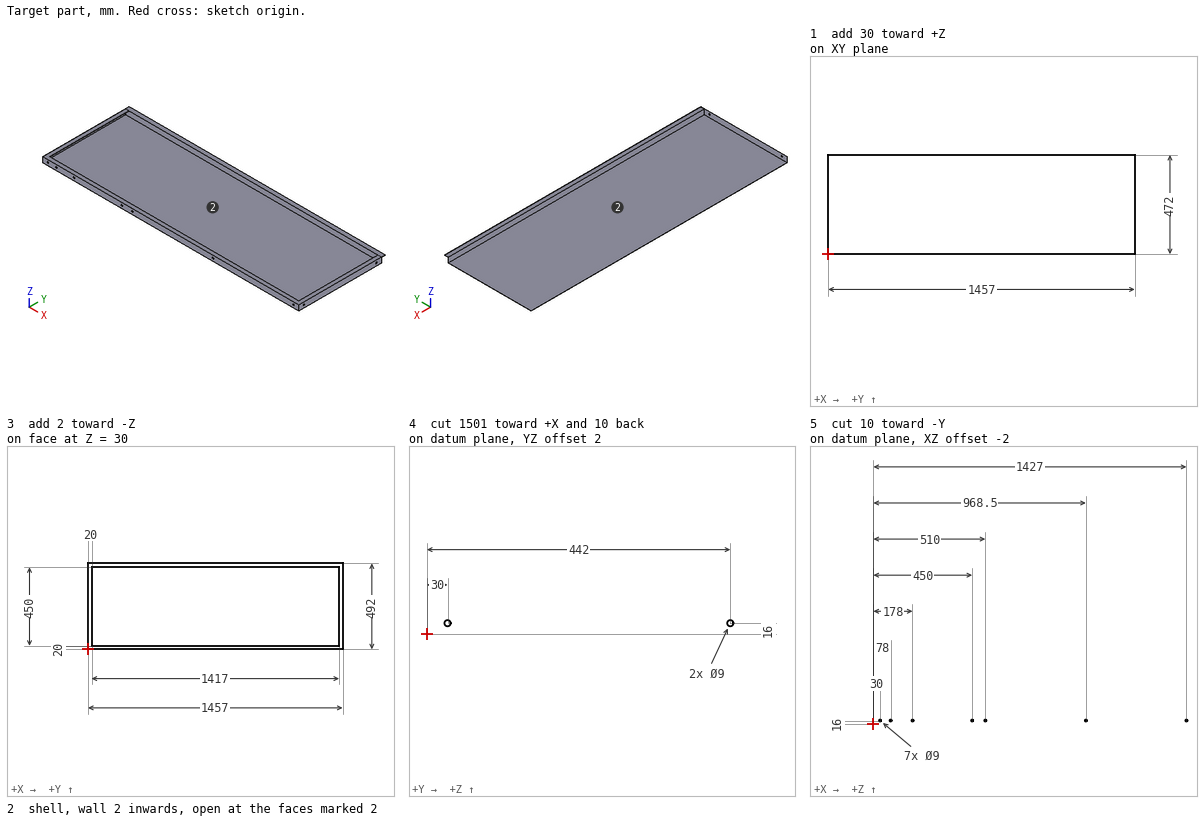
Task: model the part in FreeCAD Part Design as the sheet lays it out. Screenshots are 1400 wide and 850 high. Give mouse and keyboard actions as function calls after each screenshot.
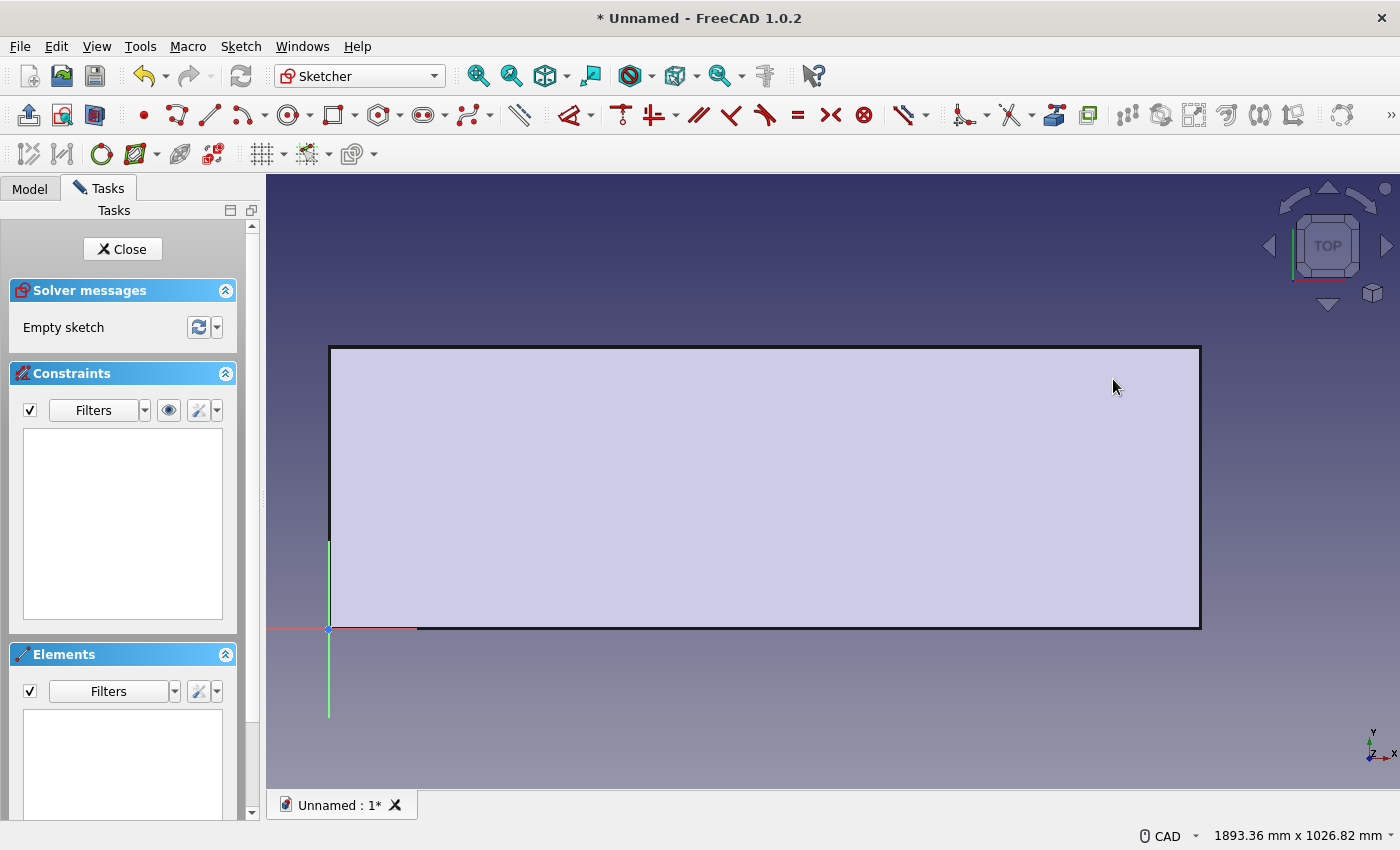
click(332, 116)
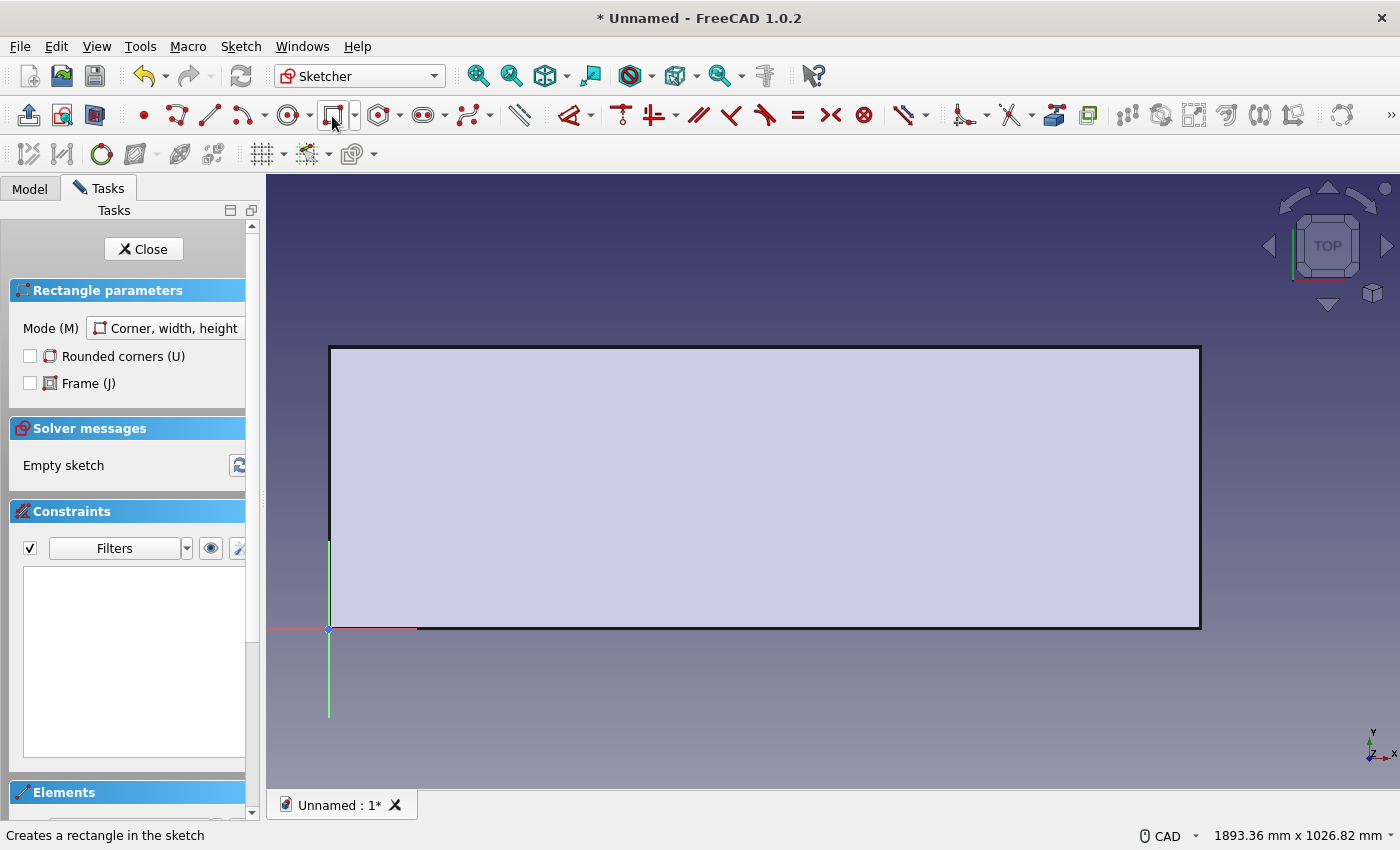
click(329, 629)
move(1201, 334)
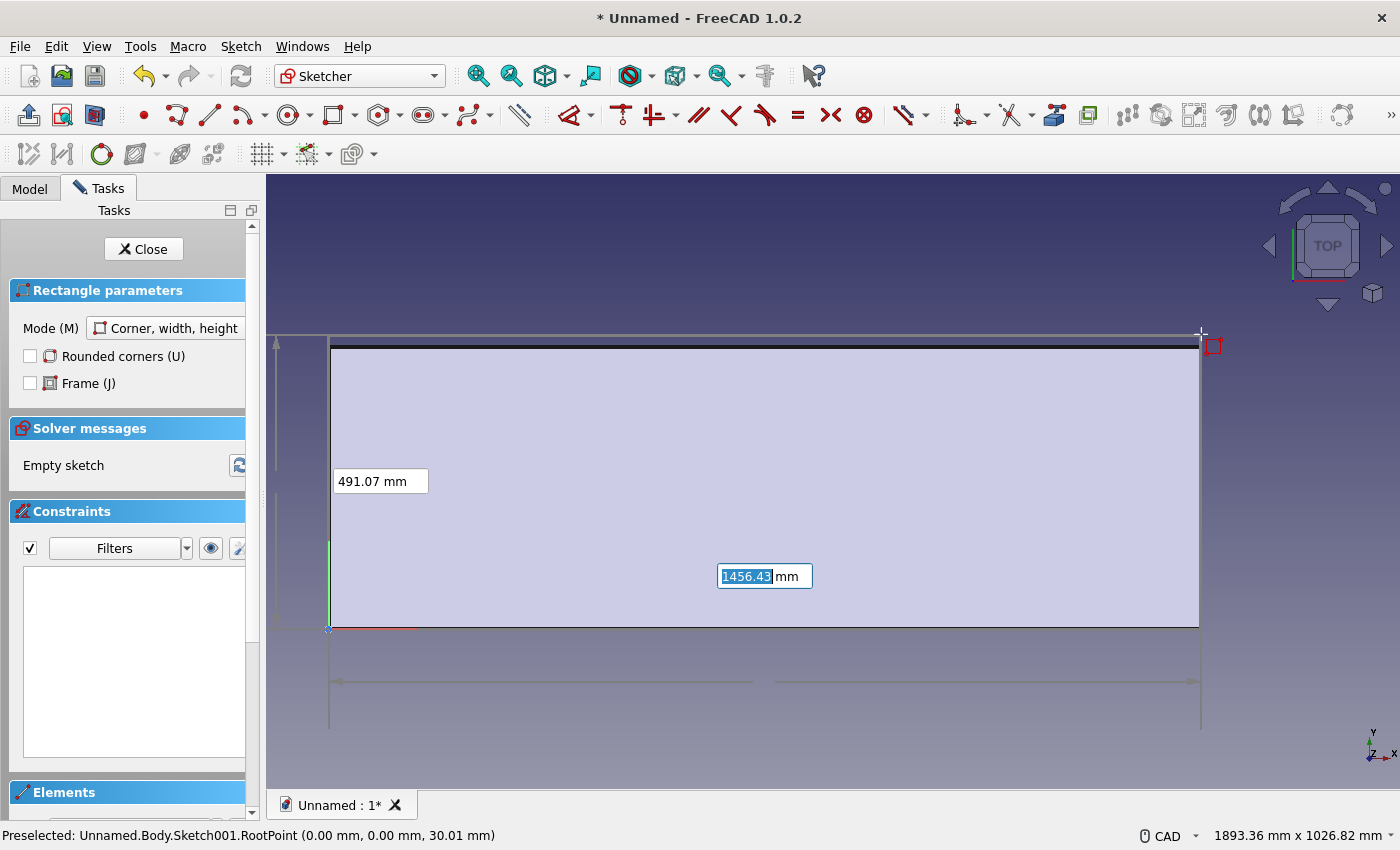
text(1457)
key(Tab)
text(492)
key(Return)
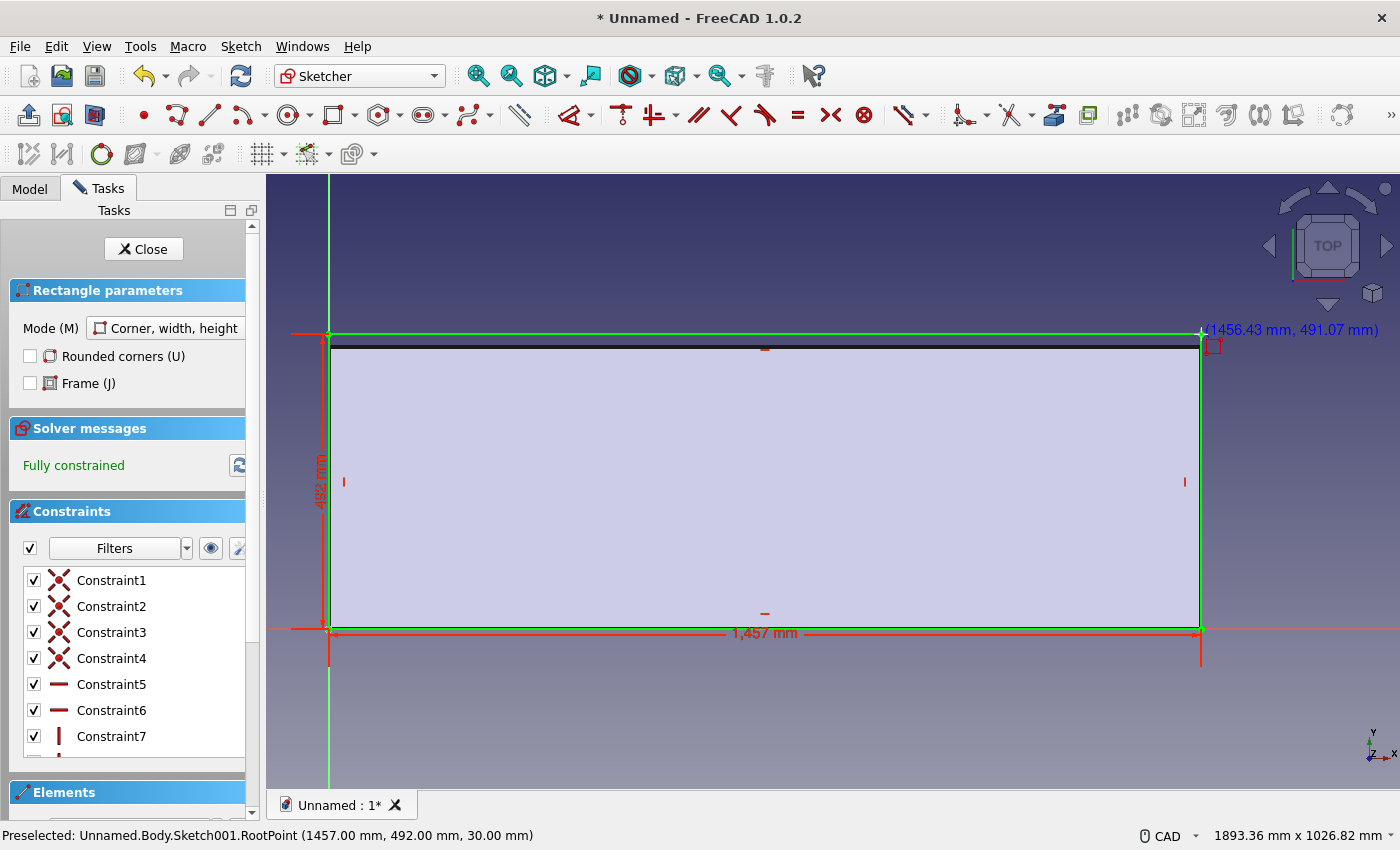
scroll(341, 348, up, 2)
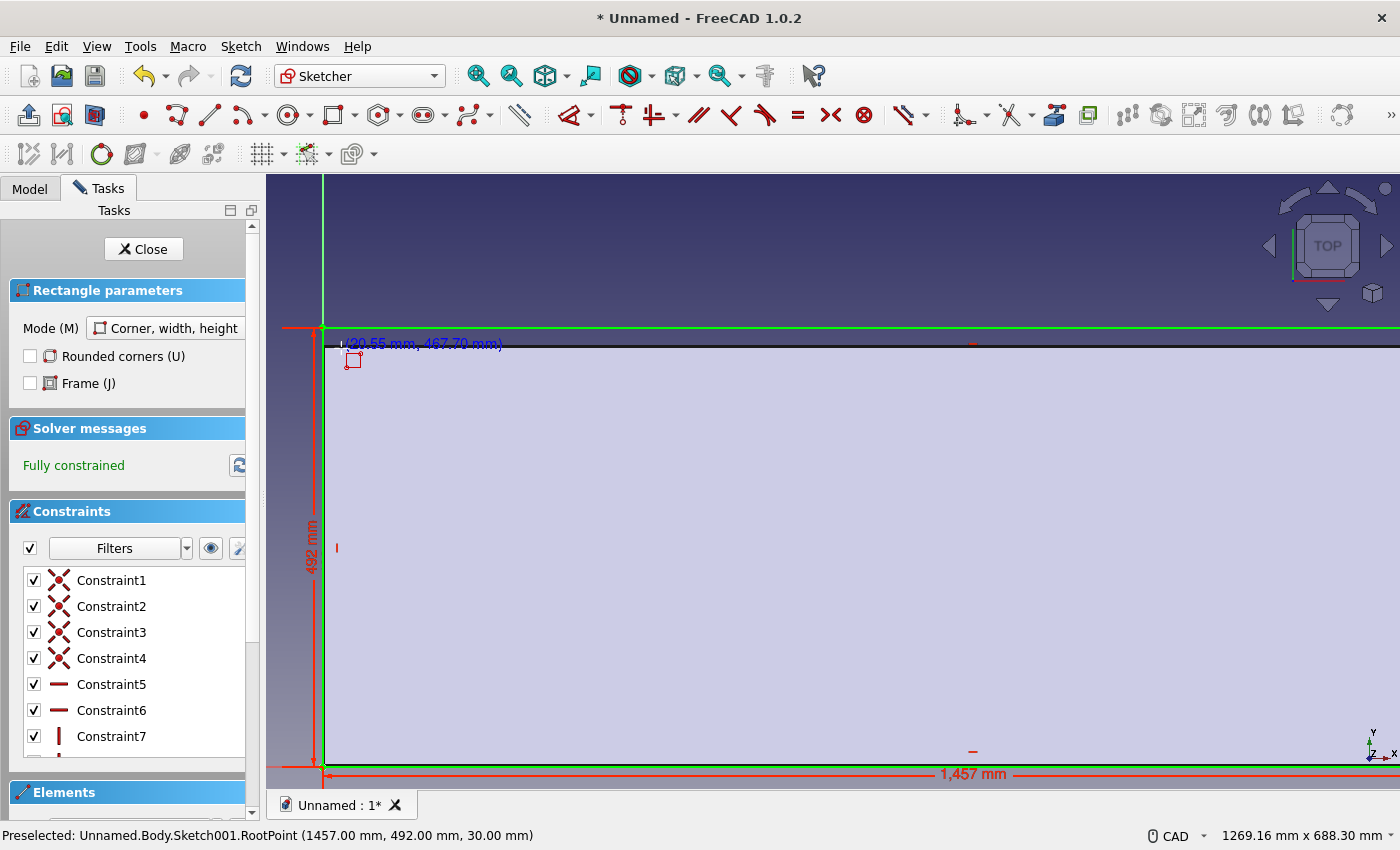
click(340, 347)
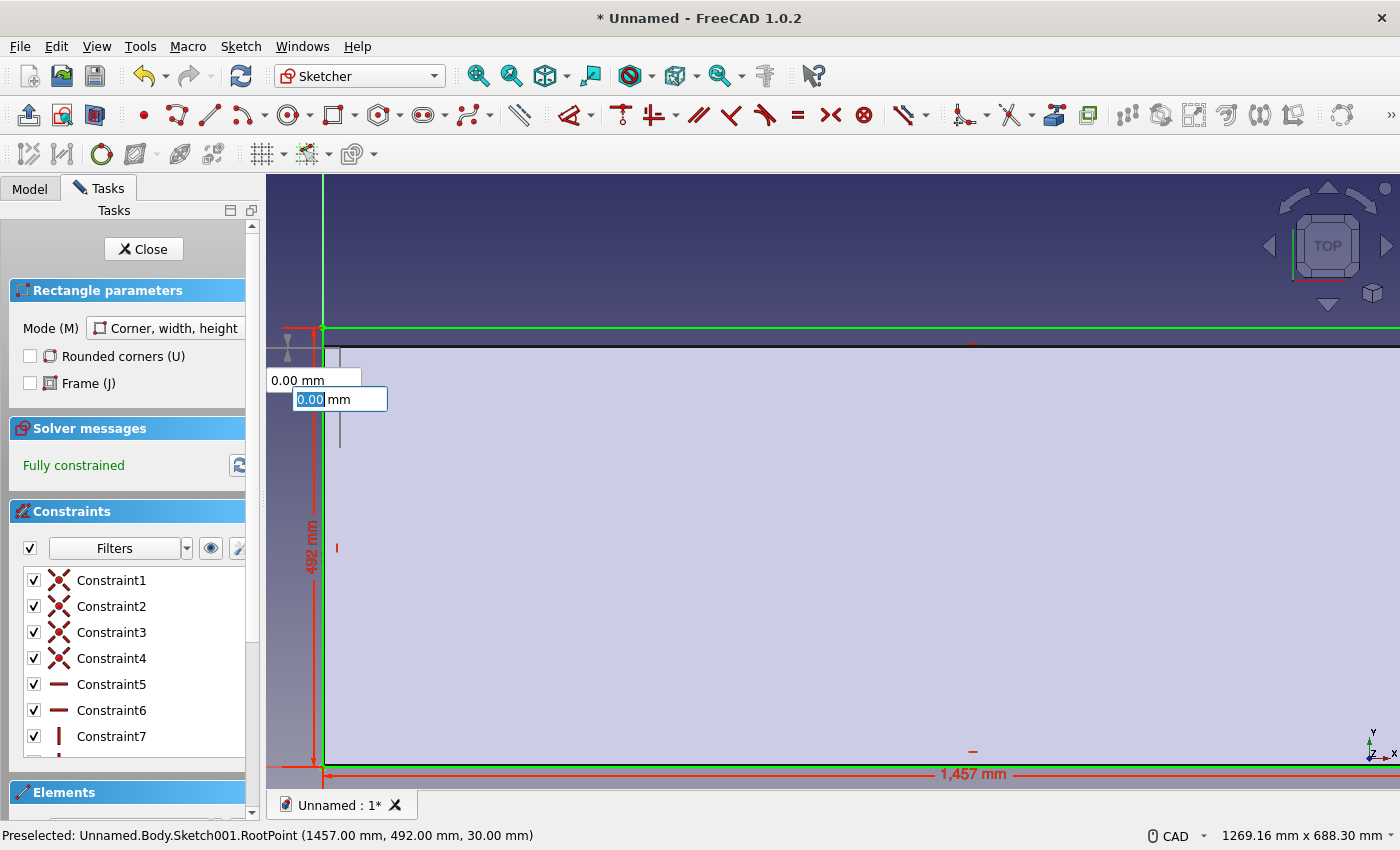
scroll(510, 401, down, 3)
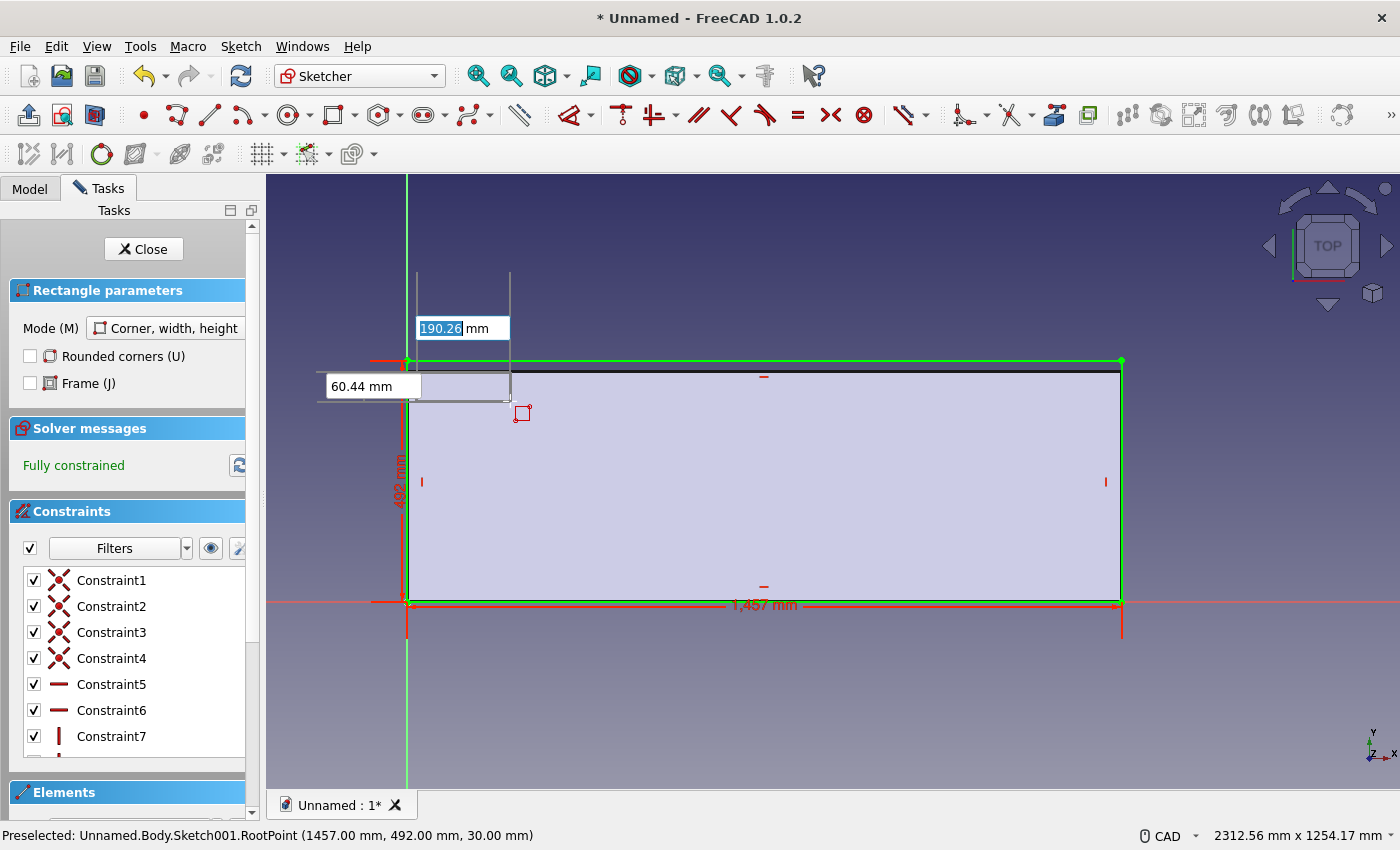
scroll(1112, 592, up, 3)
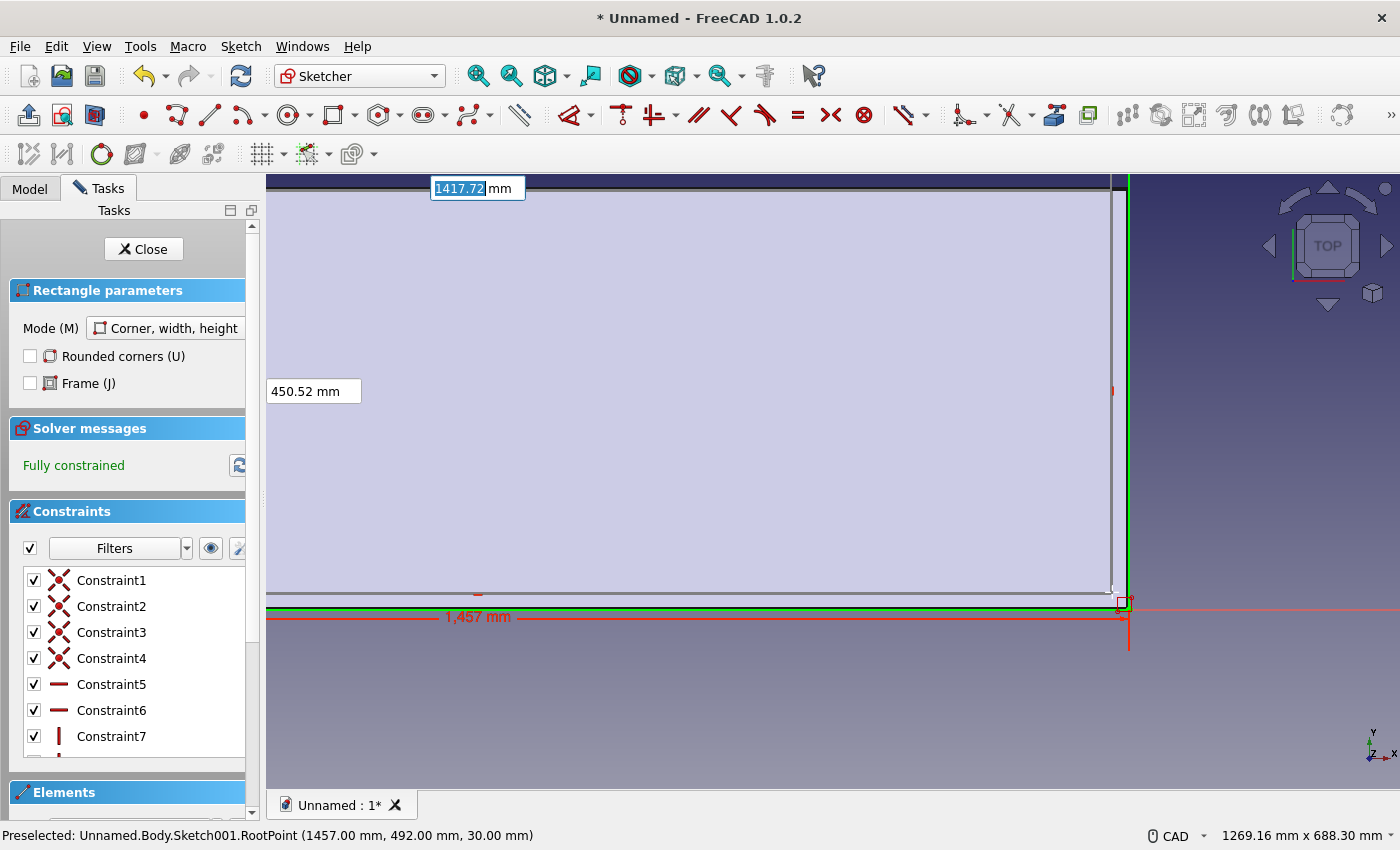
click(1111, 592)
key(Escape)